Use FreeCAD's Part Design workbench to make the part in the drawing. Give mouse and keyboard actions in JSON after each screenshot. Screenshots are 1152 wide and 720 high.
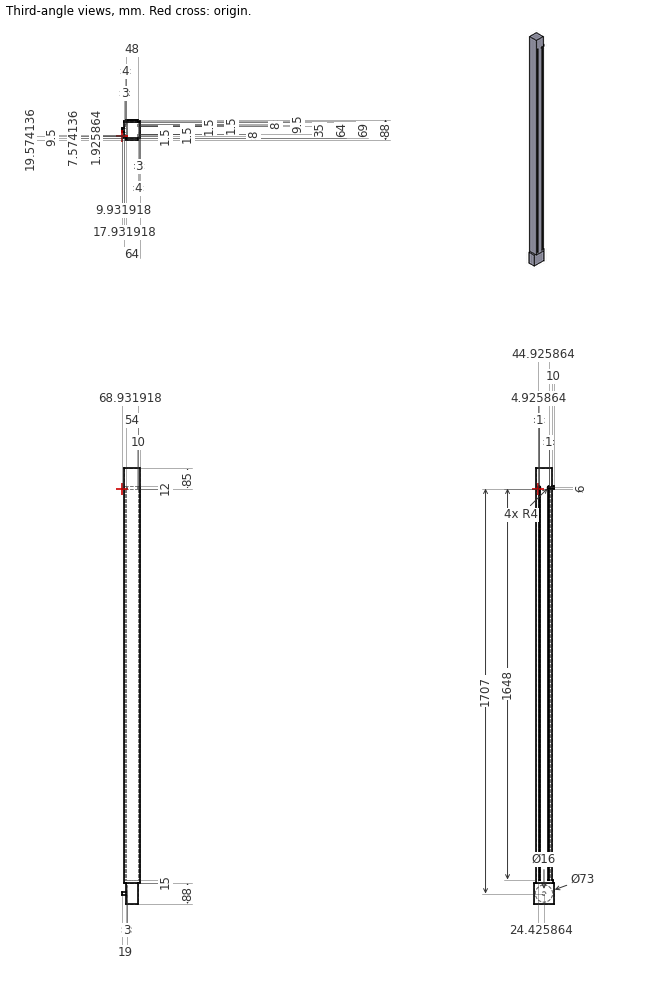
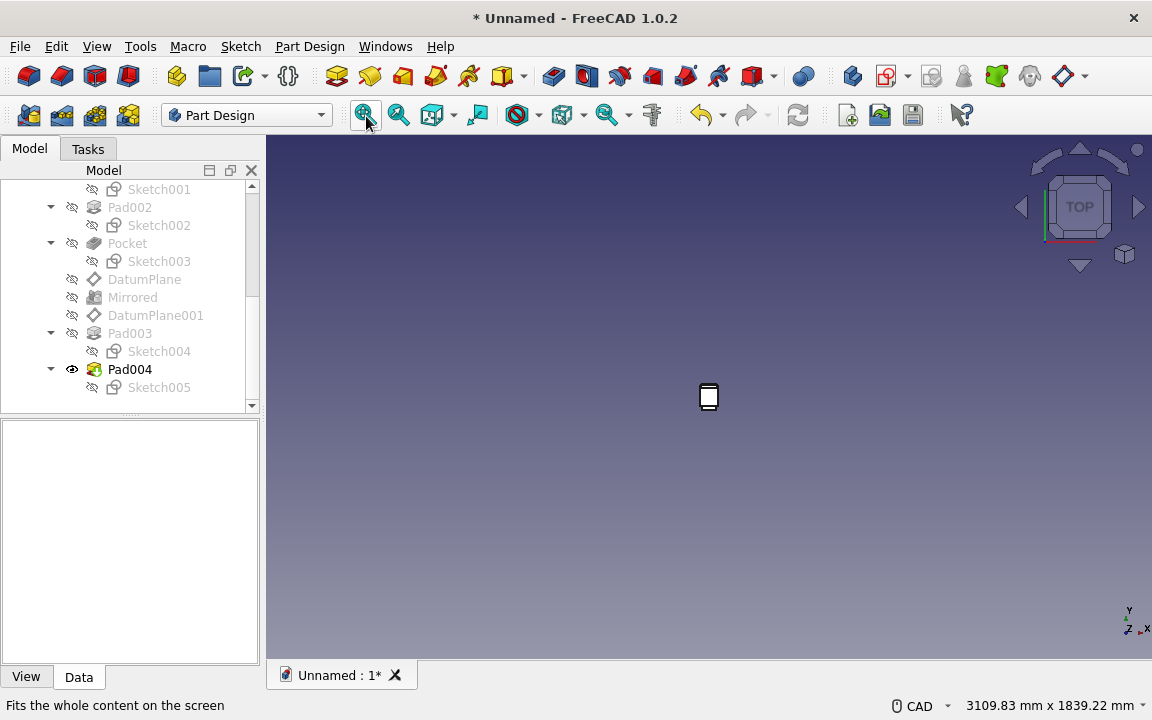
{"action": "key", "text": "1"}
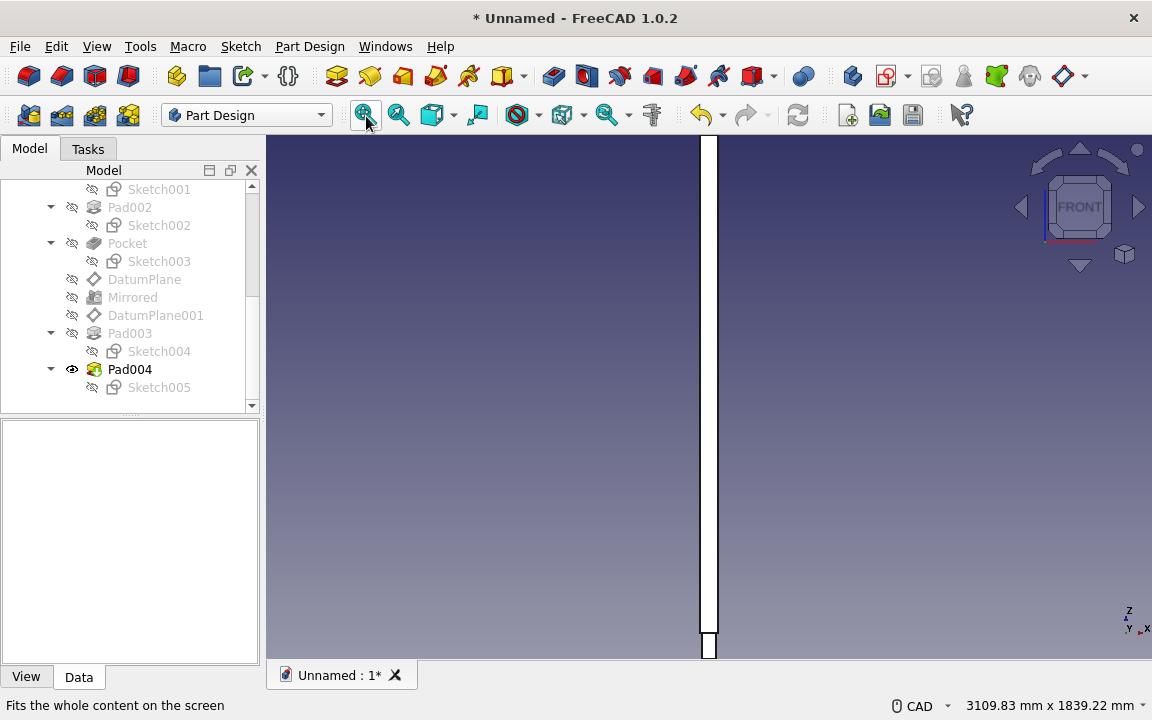
{"action": "left_click", "coordinate": [366, 116]}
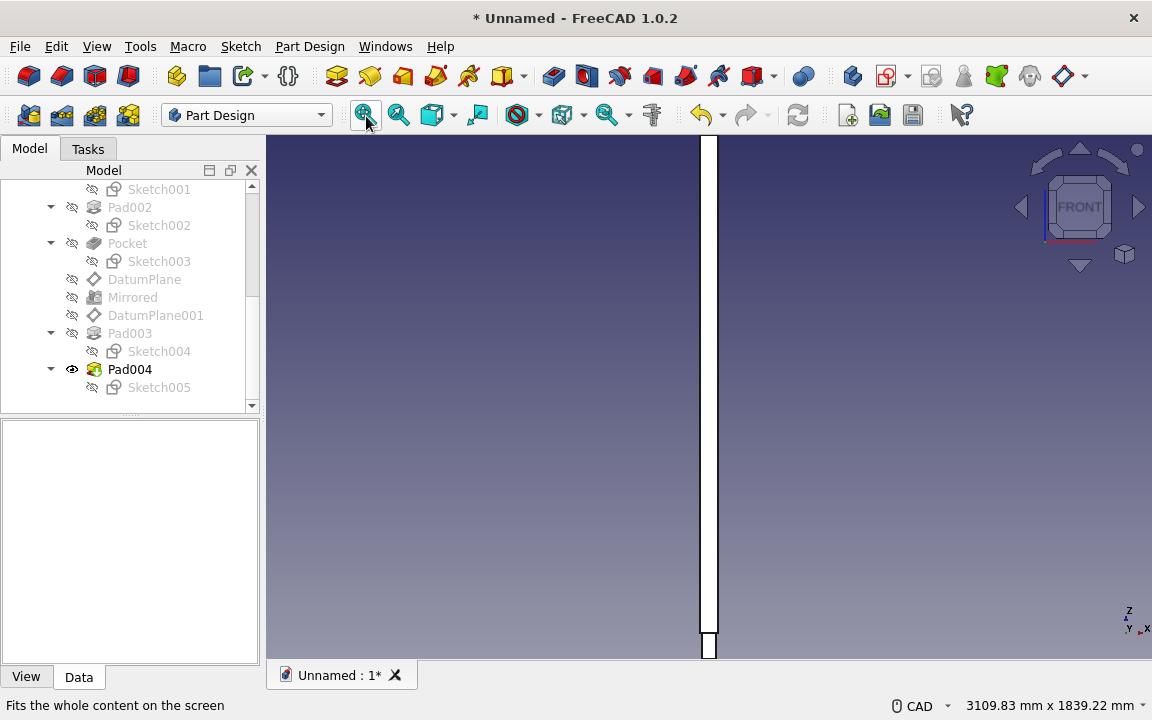
{"action": "scroll", "coordinate": [161, 293], "scroll_direction": "down", "scroll_amount": 3}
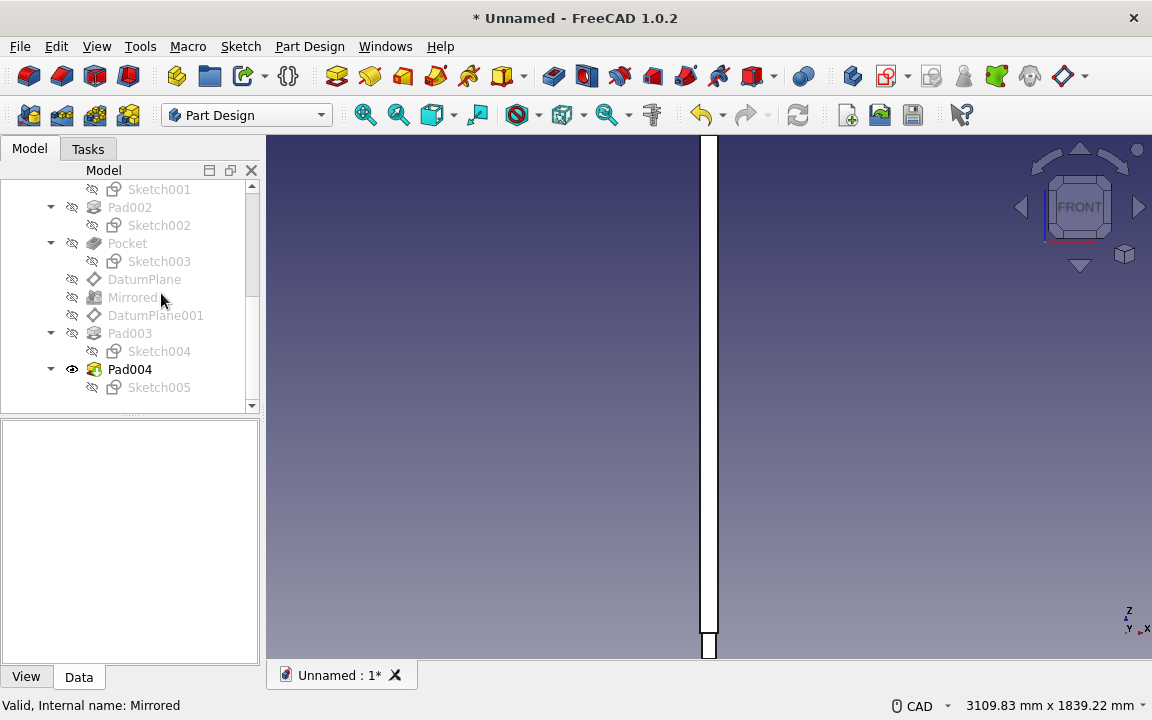
{"action": "scroll", "coordinate": [161, 293], "scroll_direction": "up", "scroll_amount": 15}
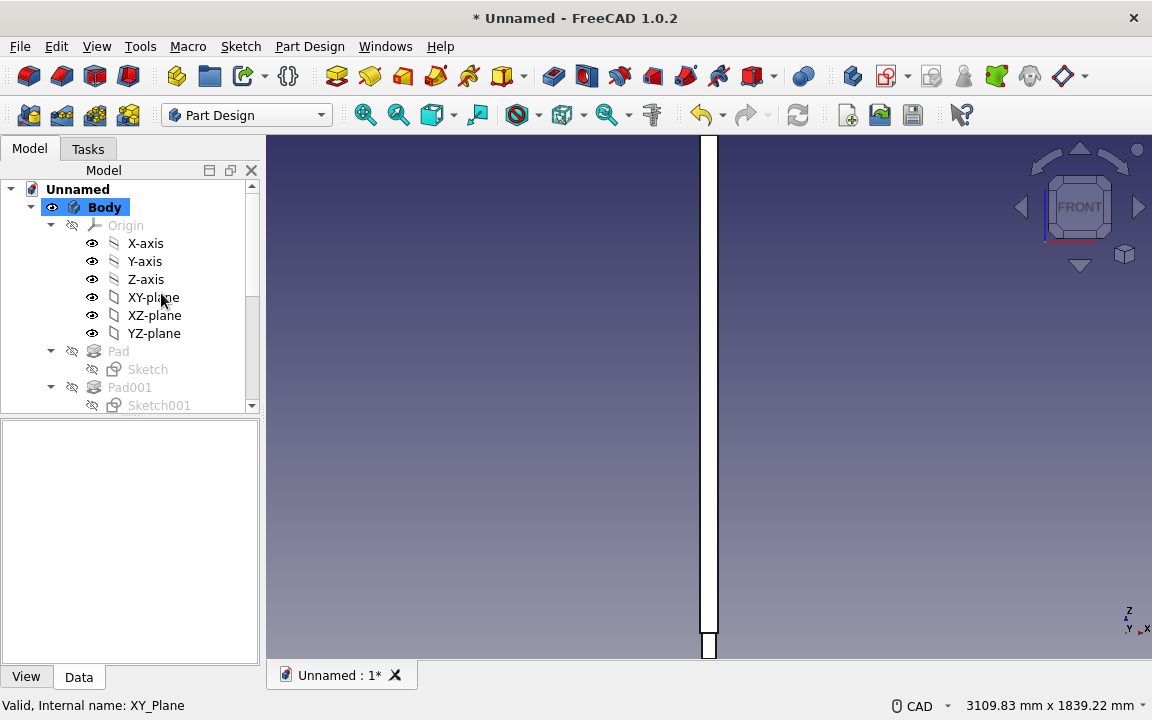
{"action": "left_click", "coordinate": [137, 333]}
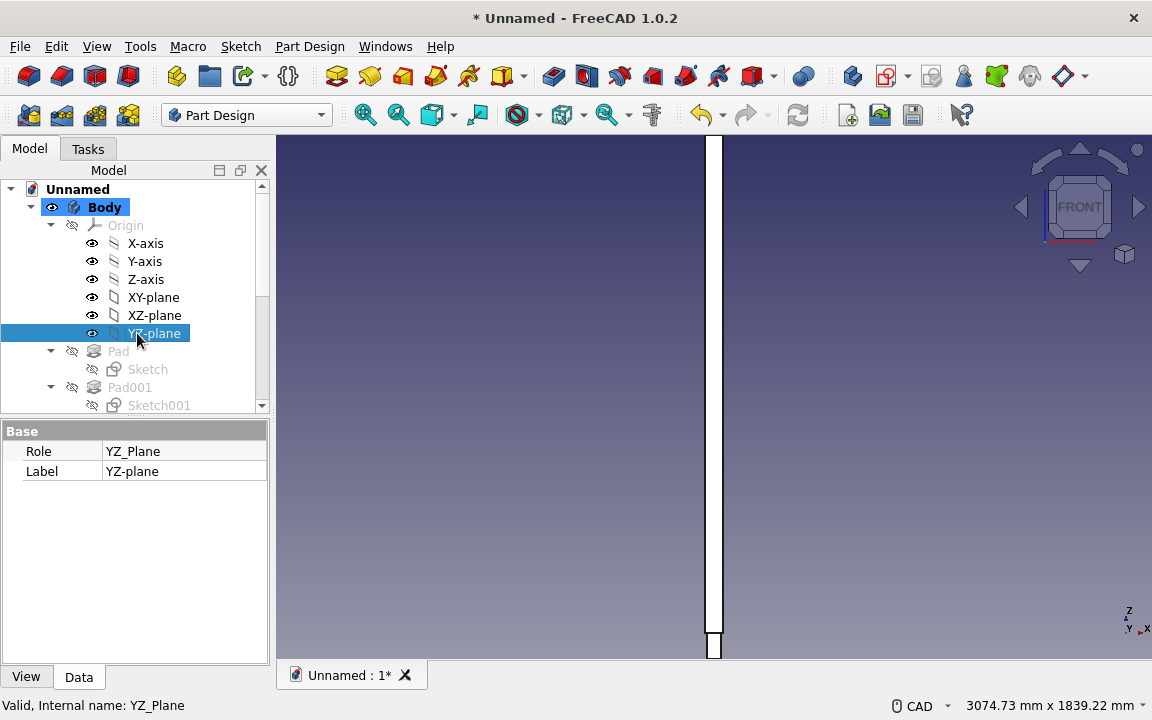
{"action": "left_click", "coordinate": [1062, 76]}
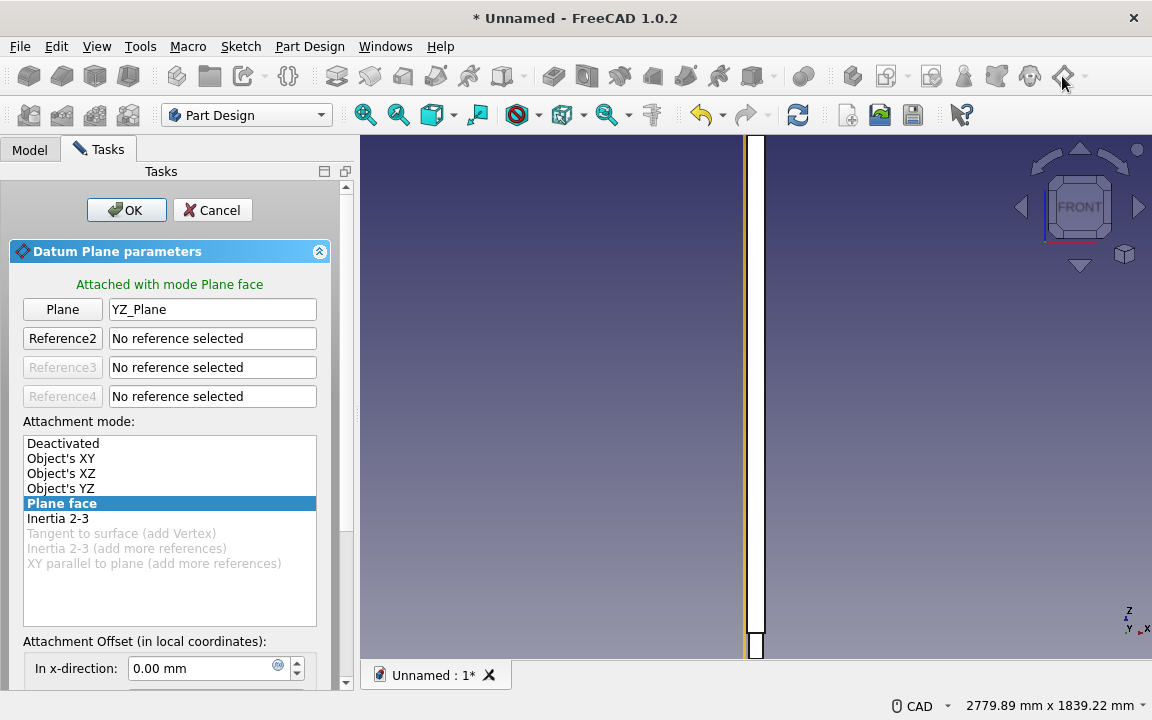
{"action": "scroll", "coordinate": [346, 436], "scroll_direction": "down", "scroll_amount": 2}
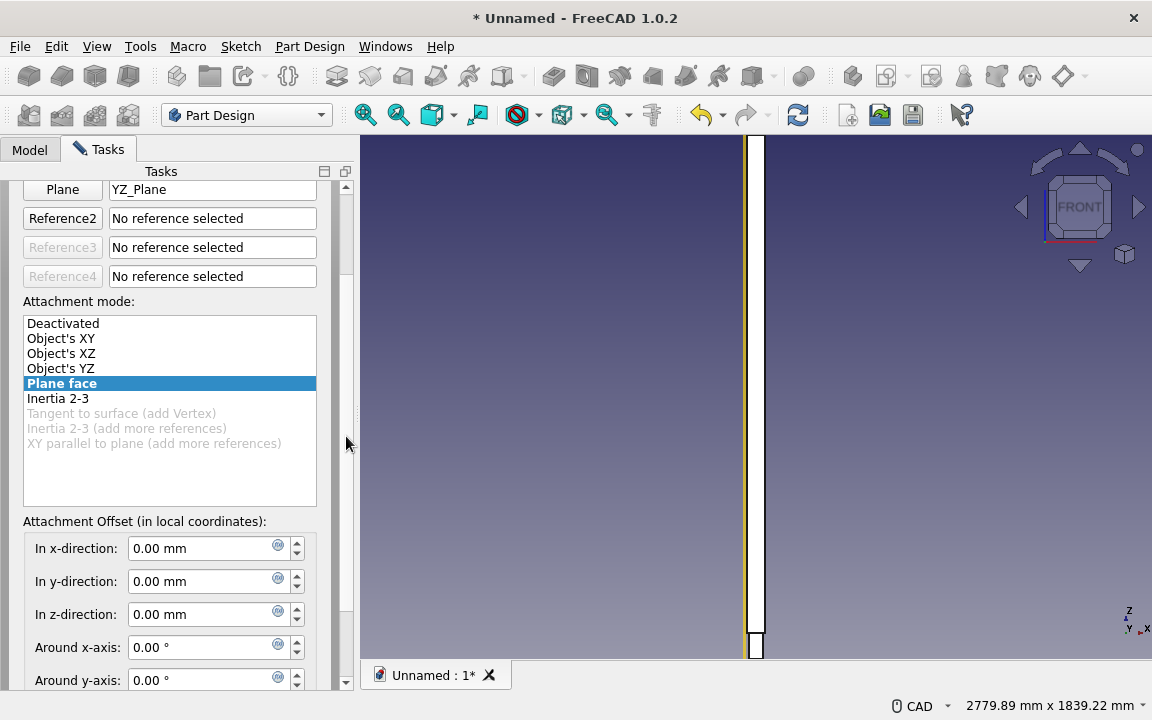
{"action": "triple_click", "coordinate": [210, 614]}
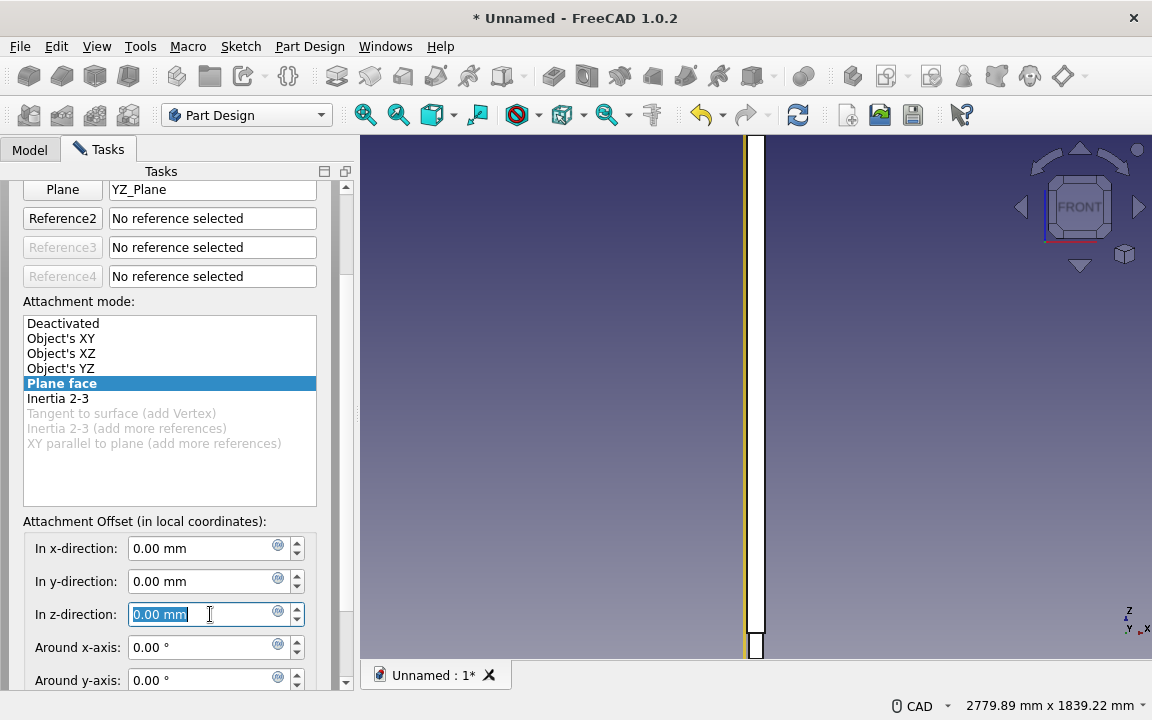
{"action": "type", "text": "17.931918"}
{"action": "key", "text": "Tab"}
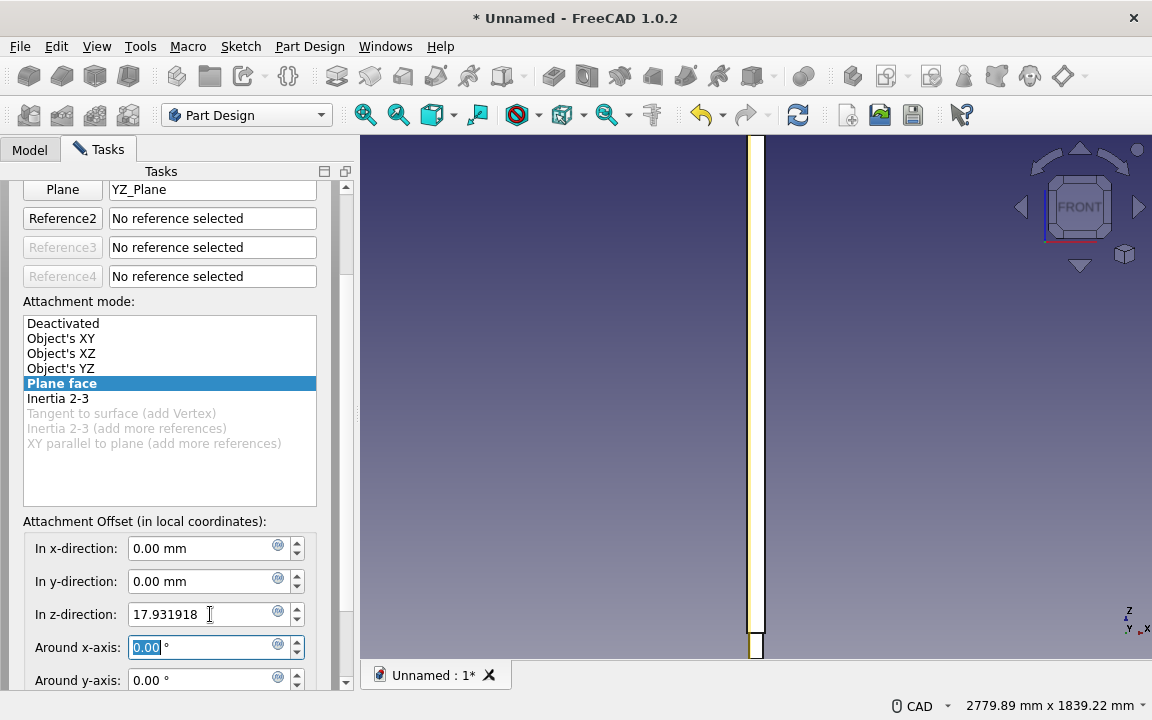
{"action": "scroll", "coordinate": [346, 436], "scroll_direction": "up", "scroll_amount": 3}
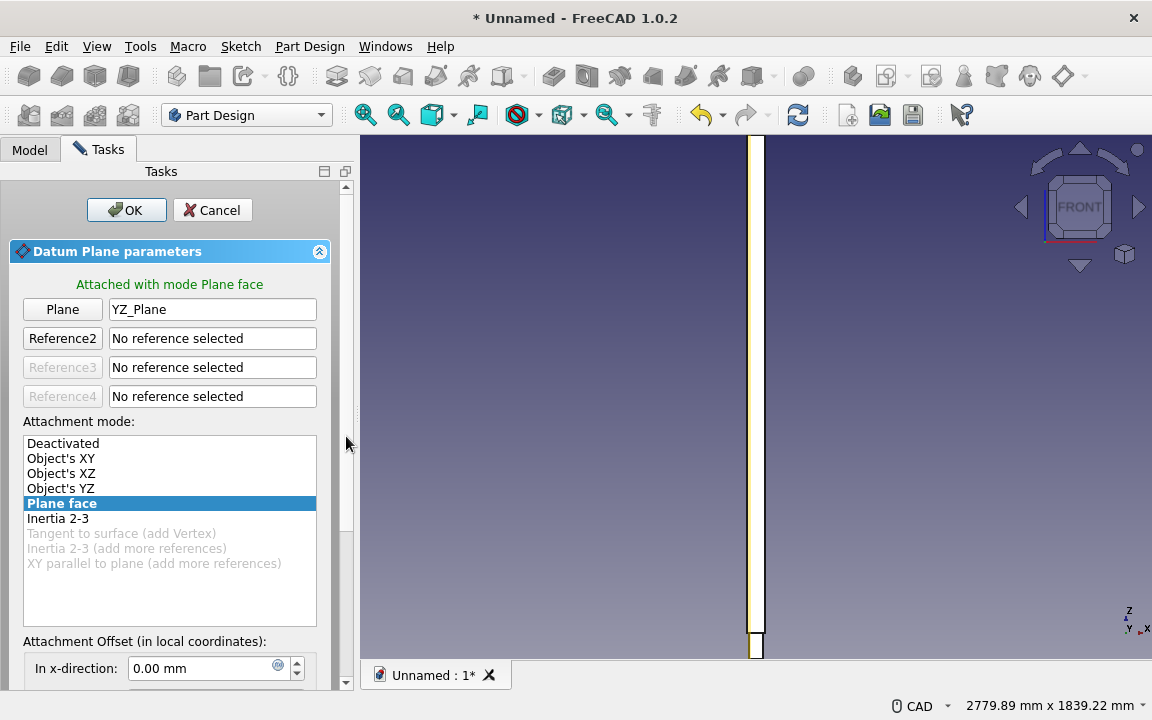
{"action": "left_click", "coordinate": [127, 210]}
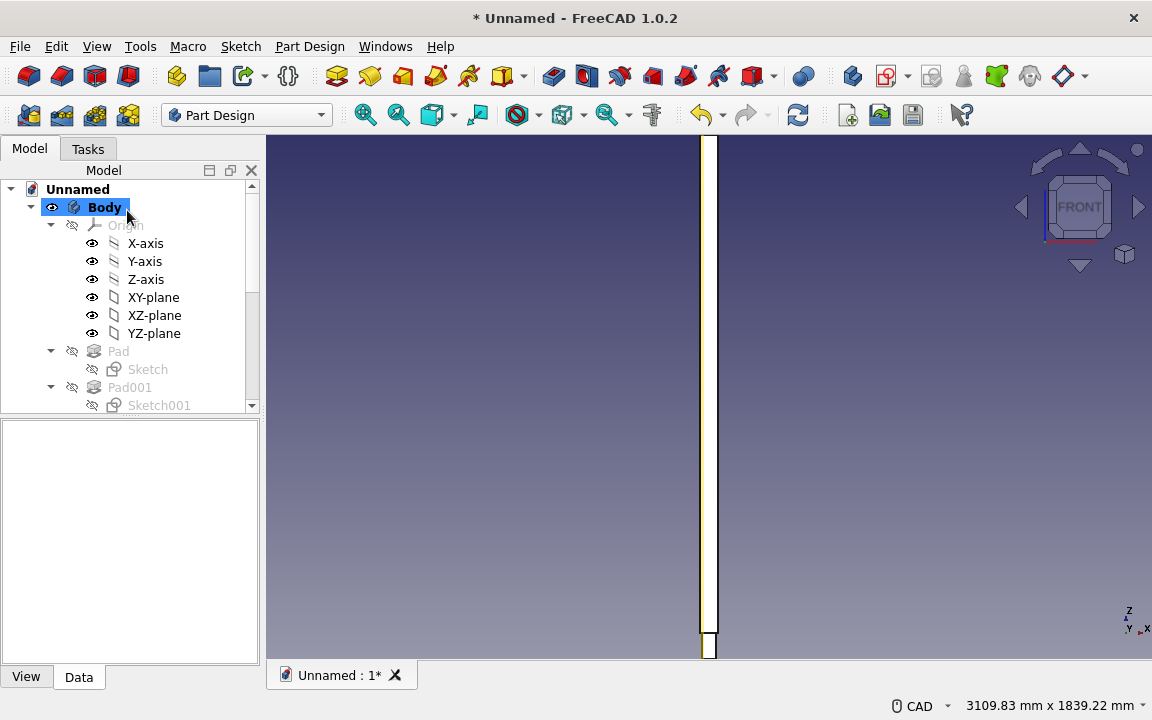
{"action": "scroll", "coordinate": [101, 293], "scroll_direction": "down", "scroll_amount": 3}